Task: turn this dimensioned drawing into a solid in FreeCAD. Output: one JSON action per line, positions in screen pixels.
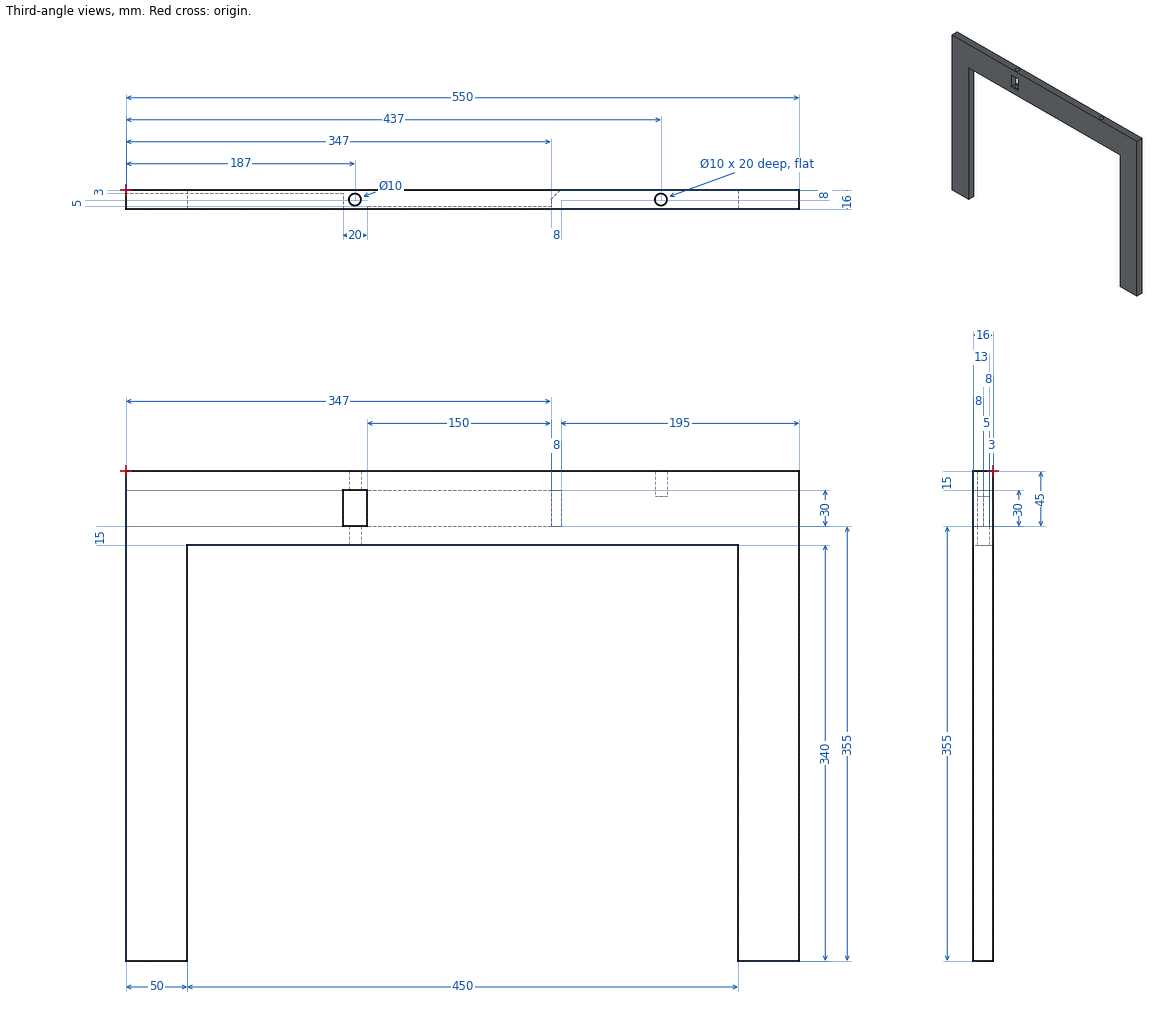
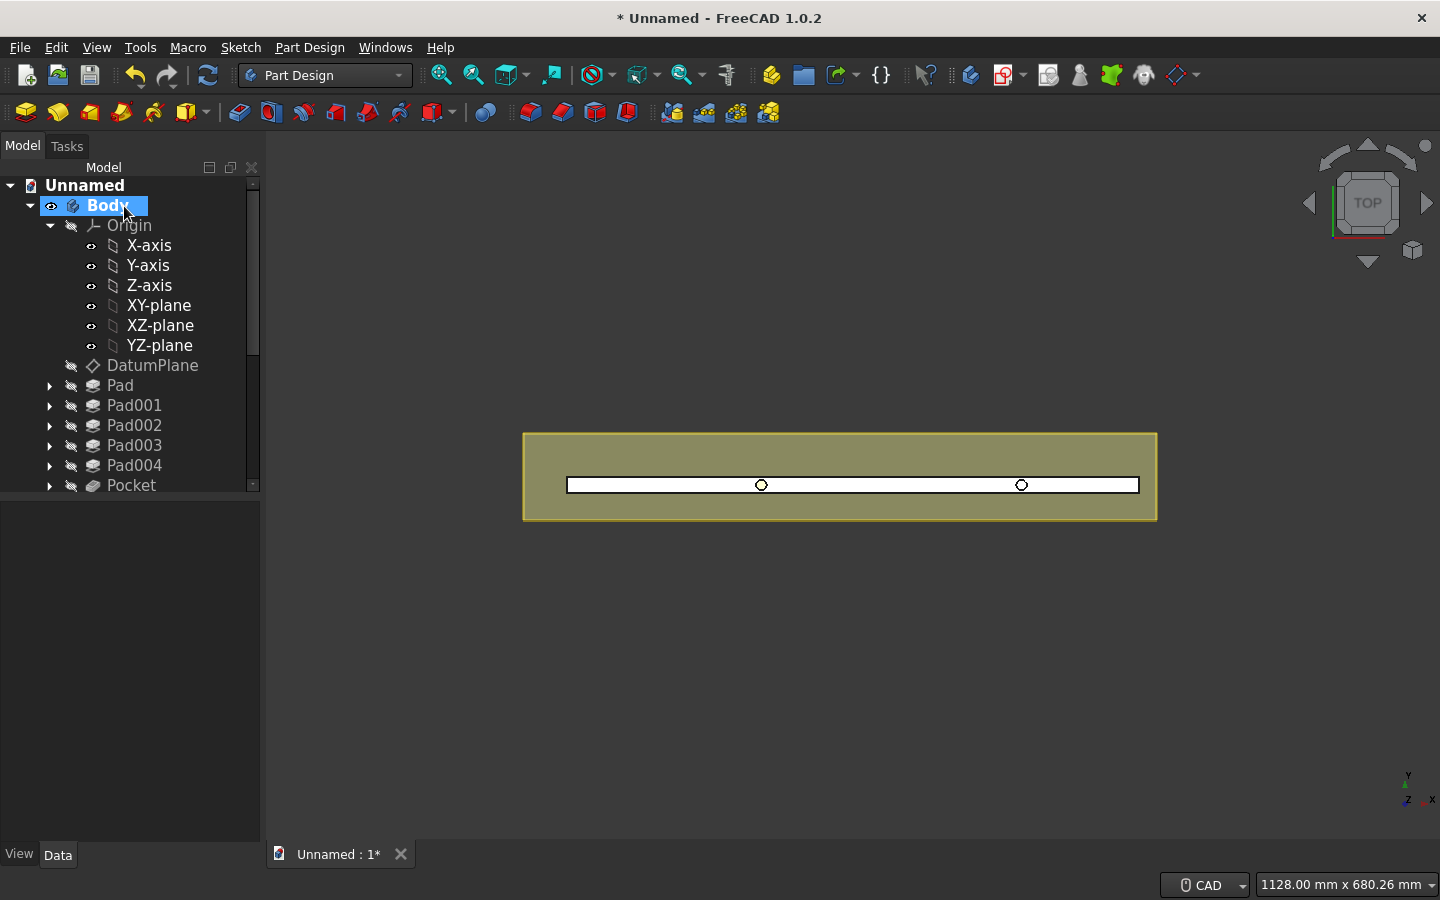
{"action": "scroll", "coordinate": [100, 341], "scroll_direction": "down", "scroll_amount": 3}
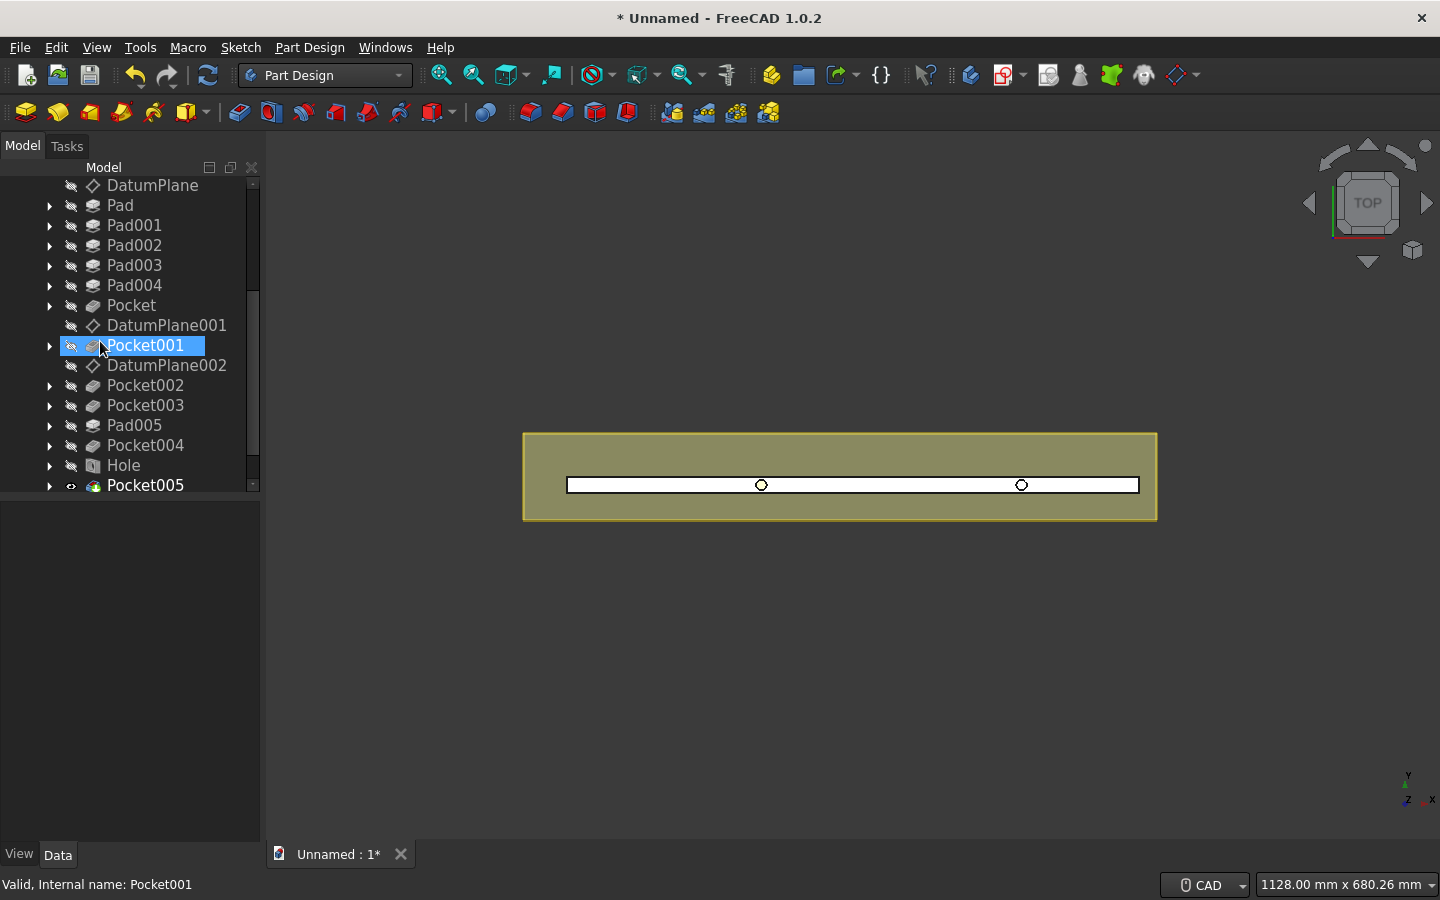
{"action": "scroll", "coordinate": [140, 341], "scroll_direction": "up", "scroll_amount": 15}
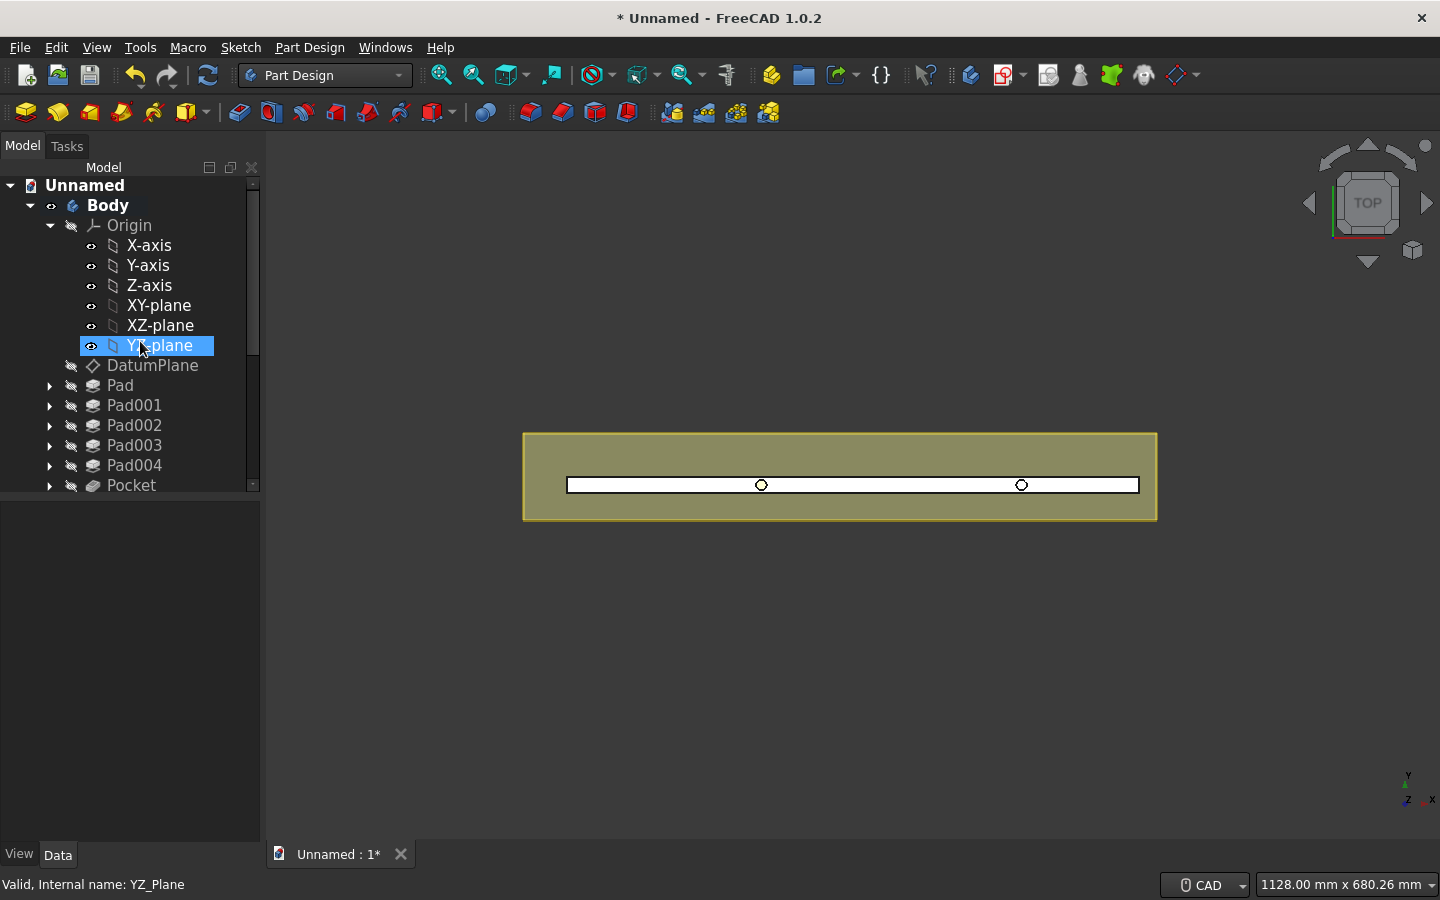
{"action": "scroll", "coordinate": [100, 341], "scroll_direction": "down", "scroll_amount": 6}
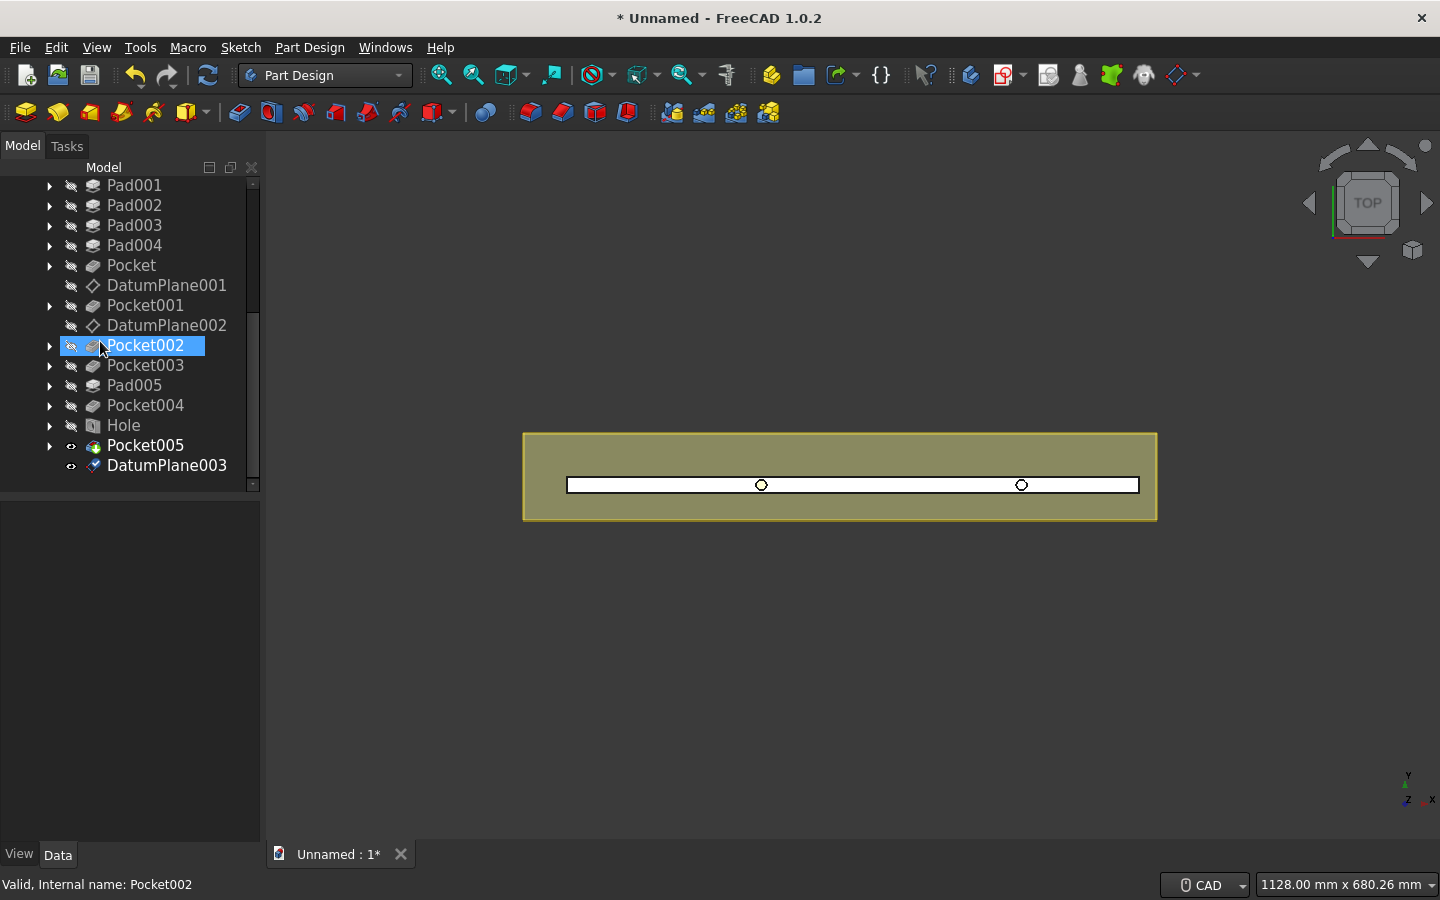
{"action": "left_click", "coordinate": [116, 466]}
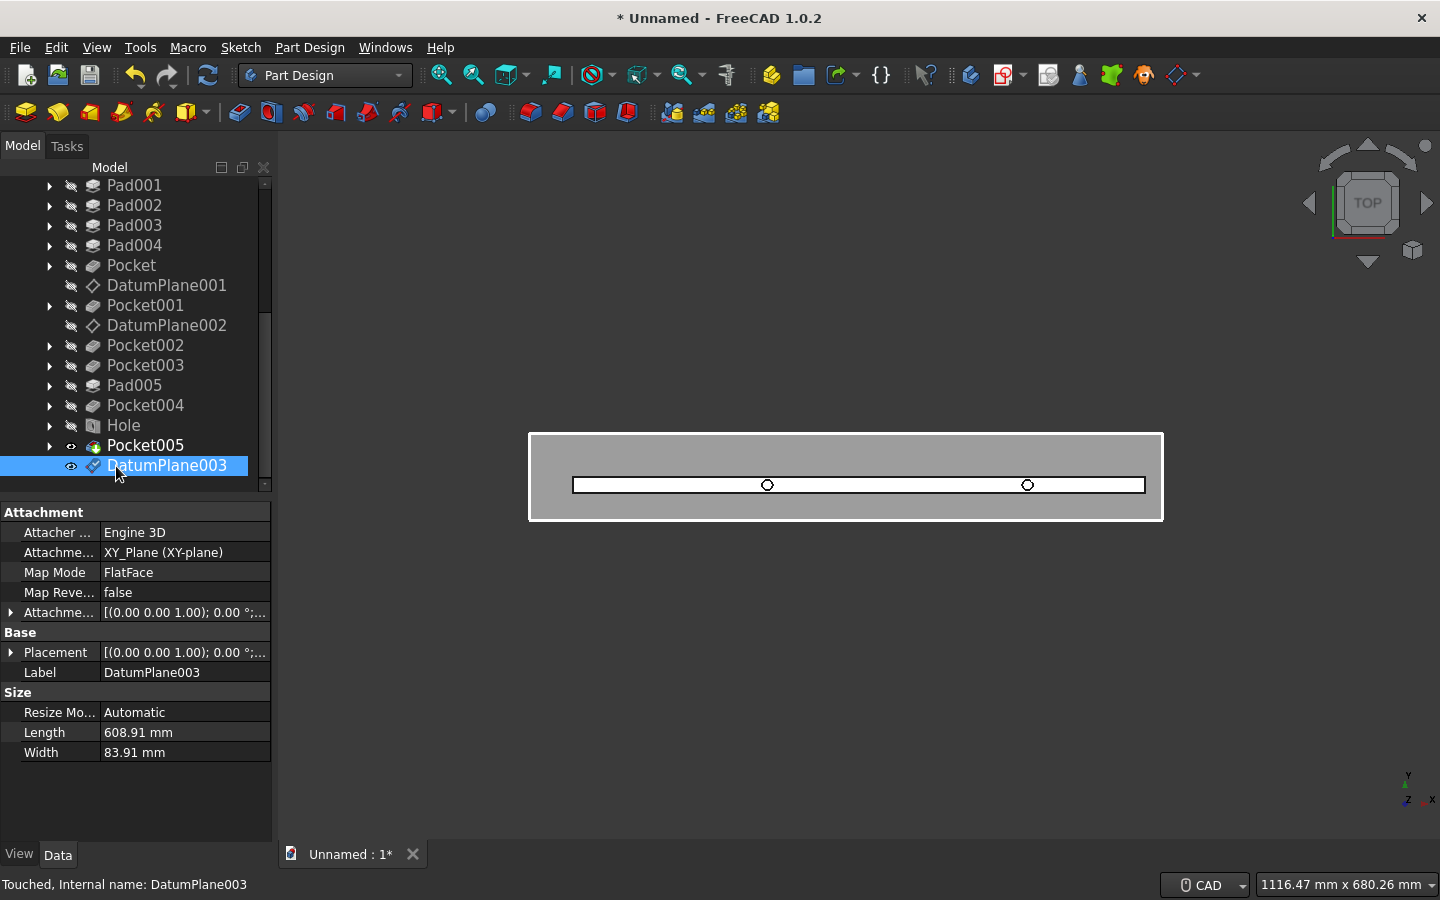
{"action": "left_click", "coordinate": [1004, 76]}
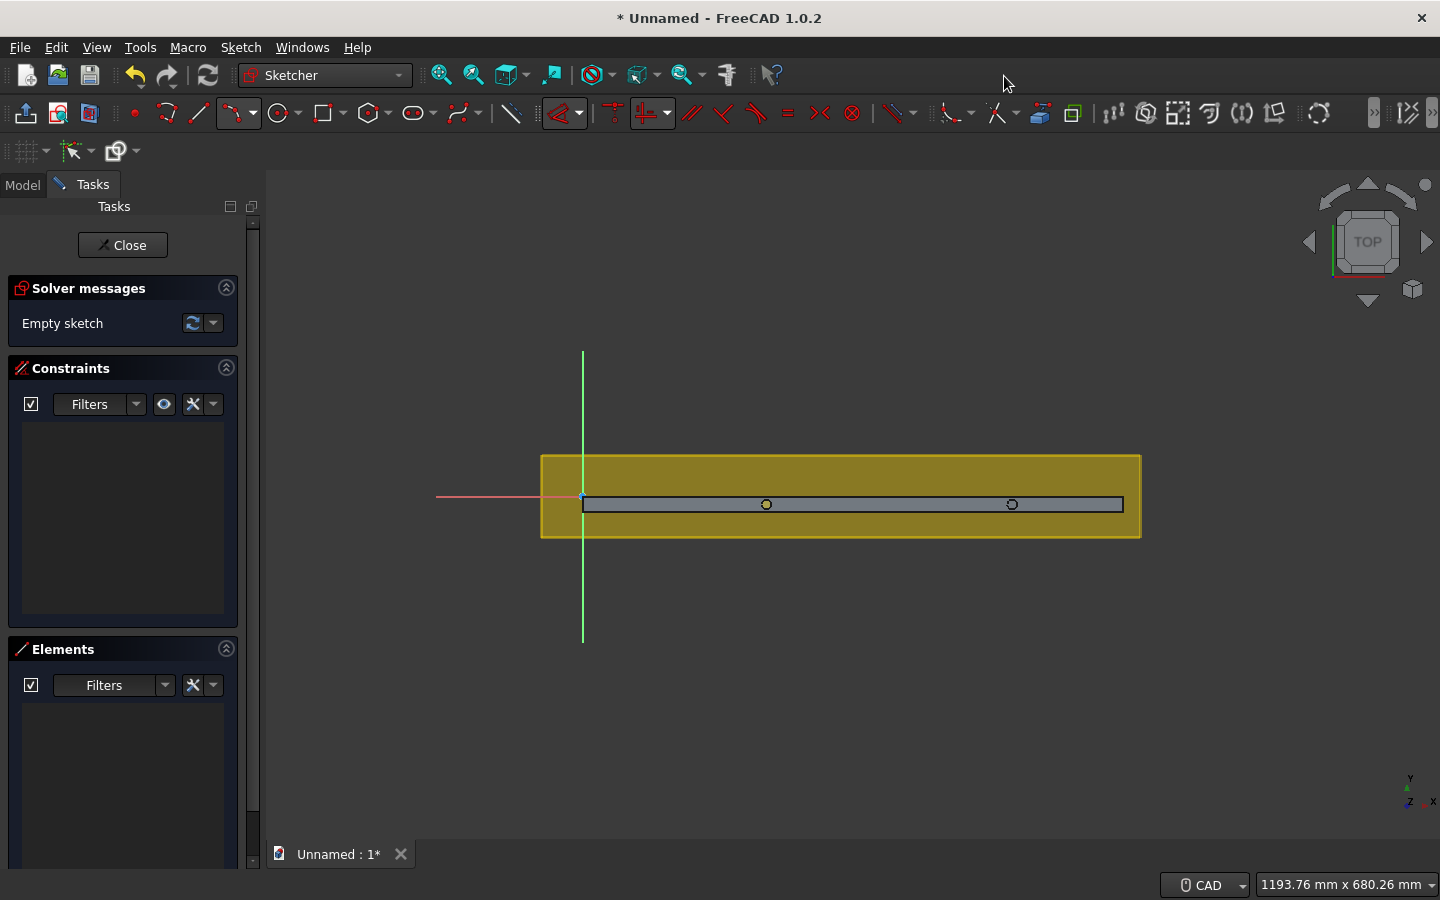
{"action": "left_click", "coordinate": [90, 114]}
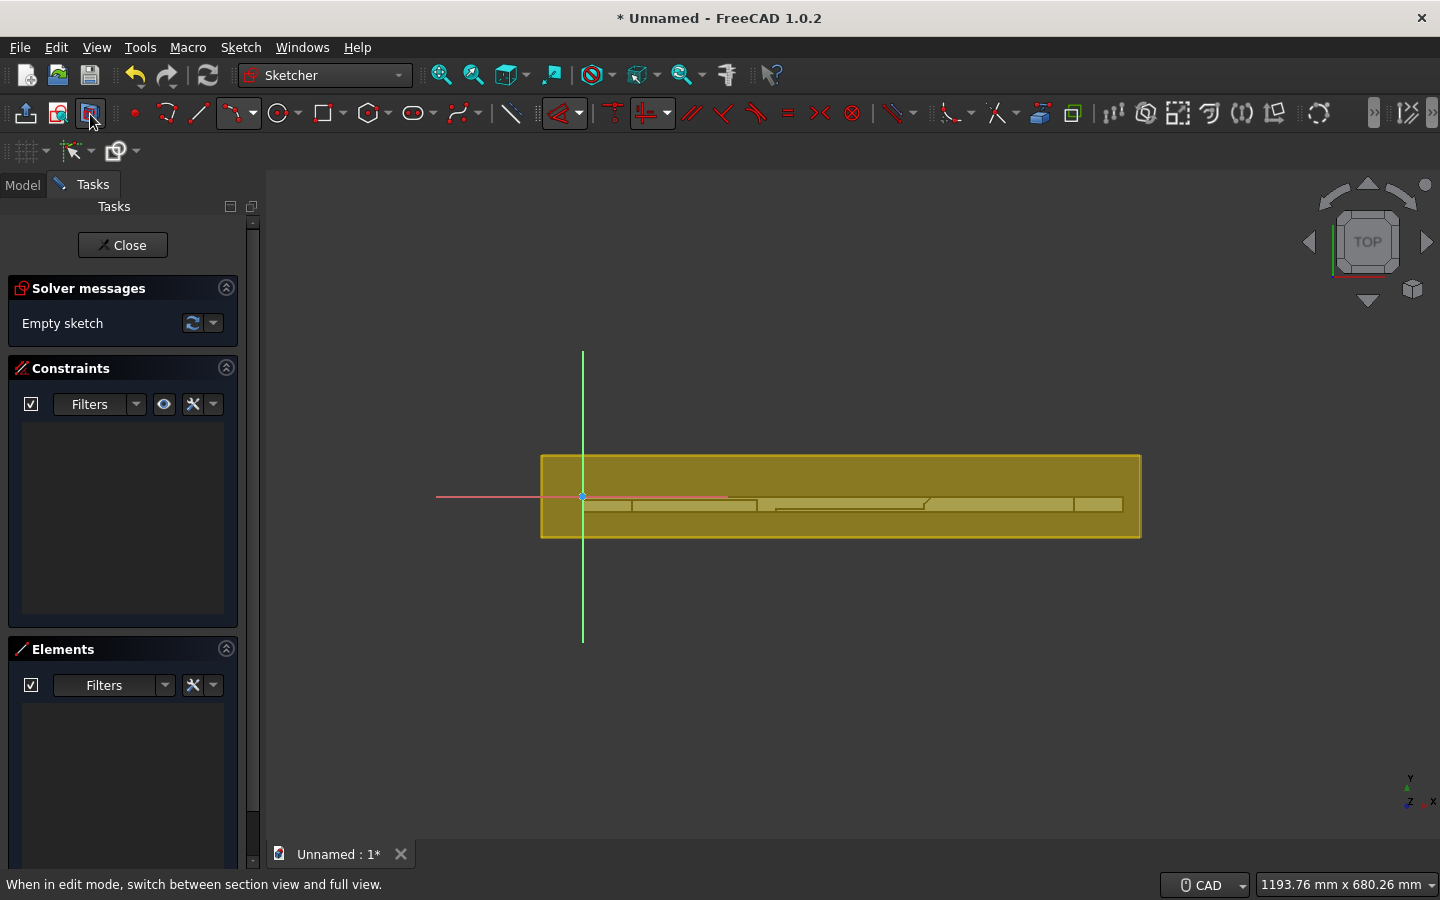
{"action": "scroll", "coordinate": [766, 504], "scroll_direction": "up", "scroll_amount": 15}